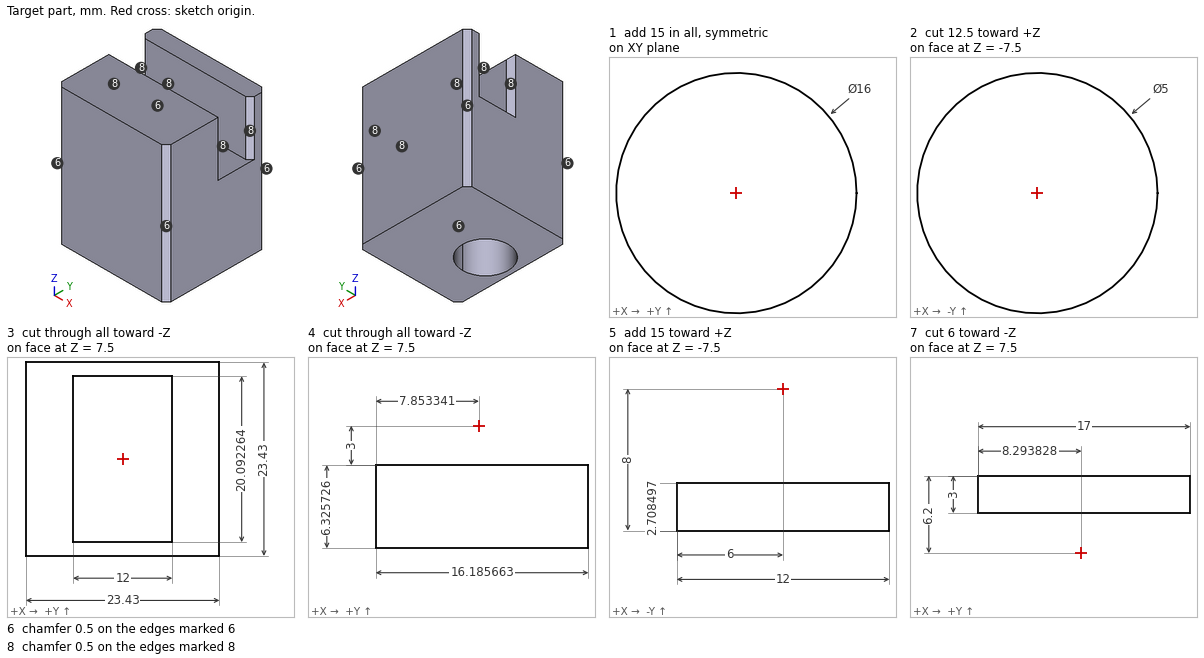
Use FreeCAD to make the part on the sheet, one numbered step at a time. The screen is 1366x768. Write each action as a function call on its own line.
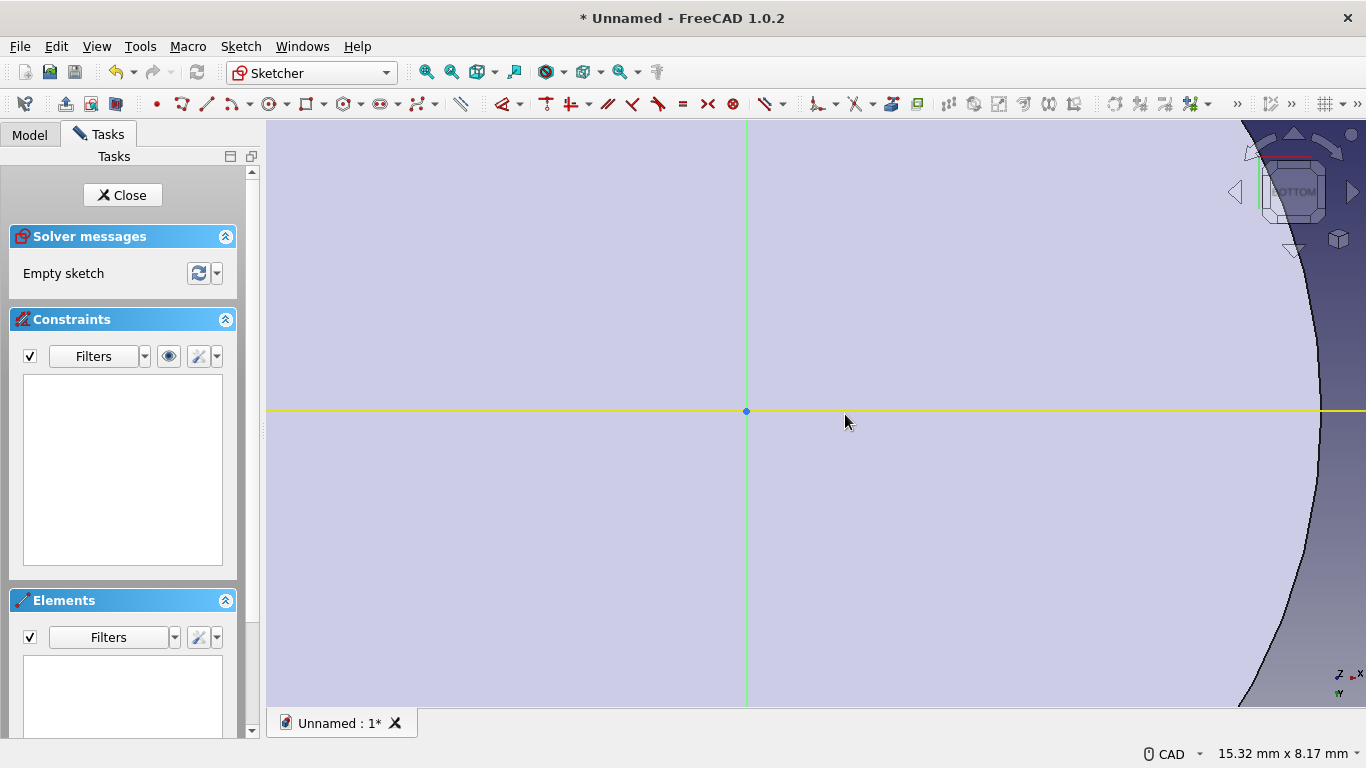
click(268, 104)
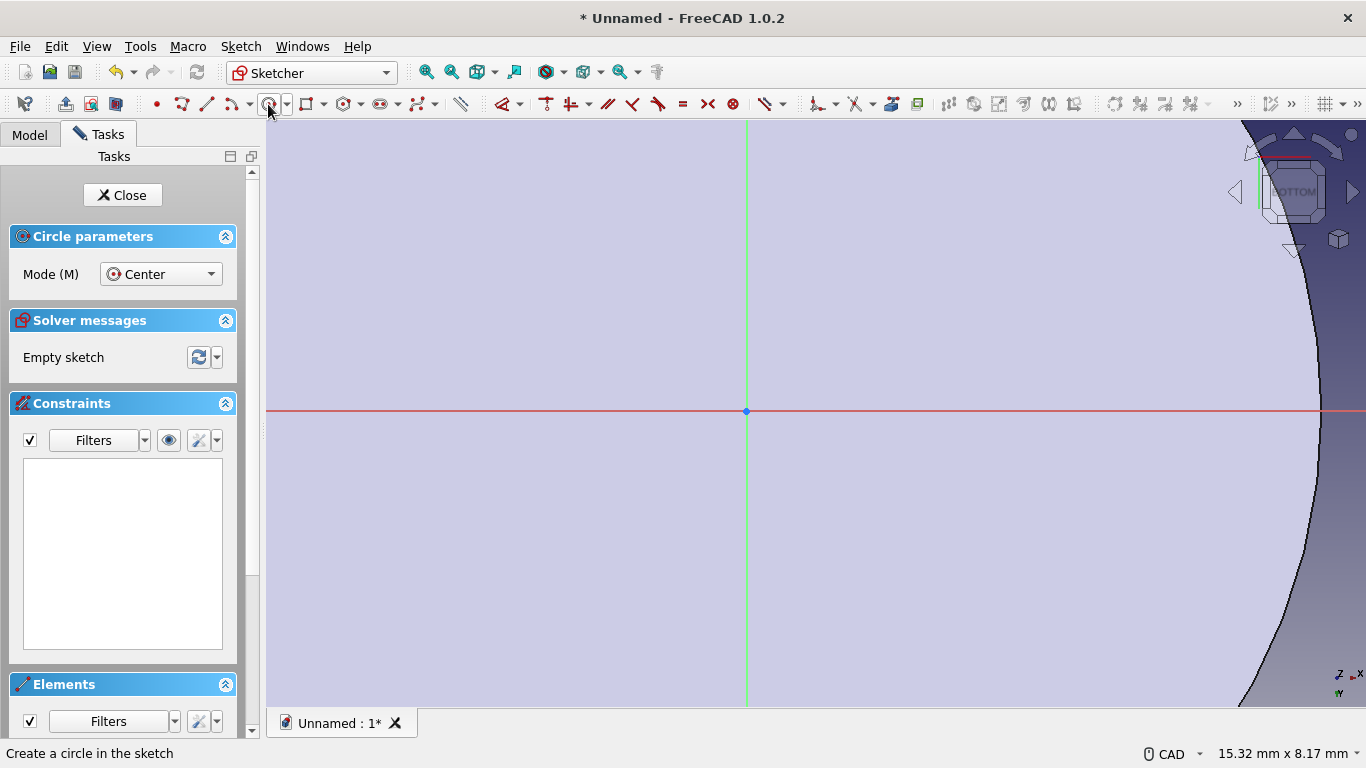
click(747, 411)
click(874, 284)
key(Escape)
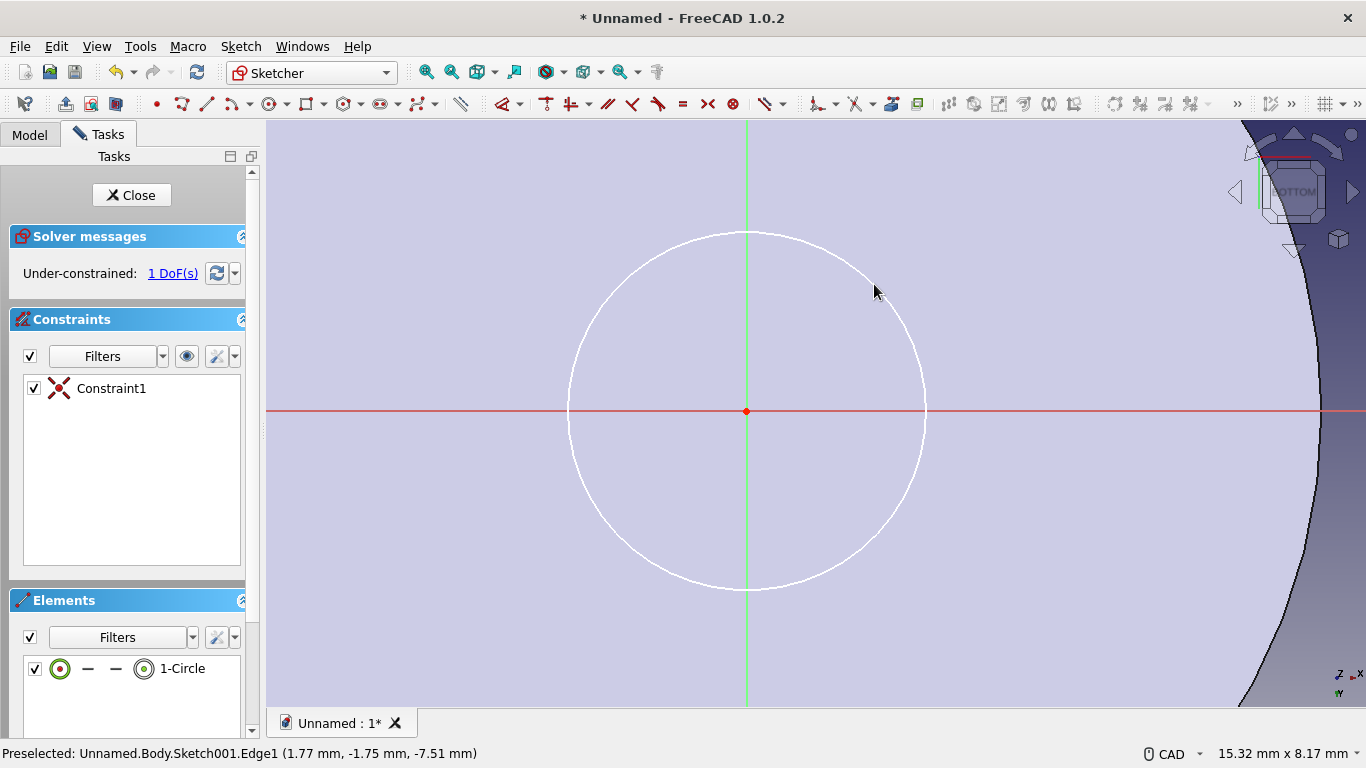
click(502, 104)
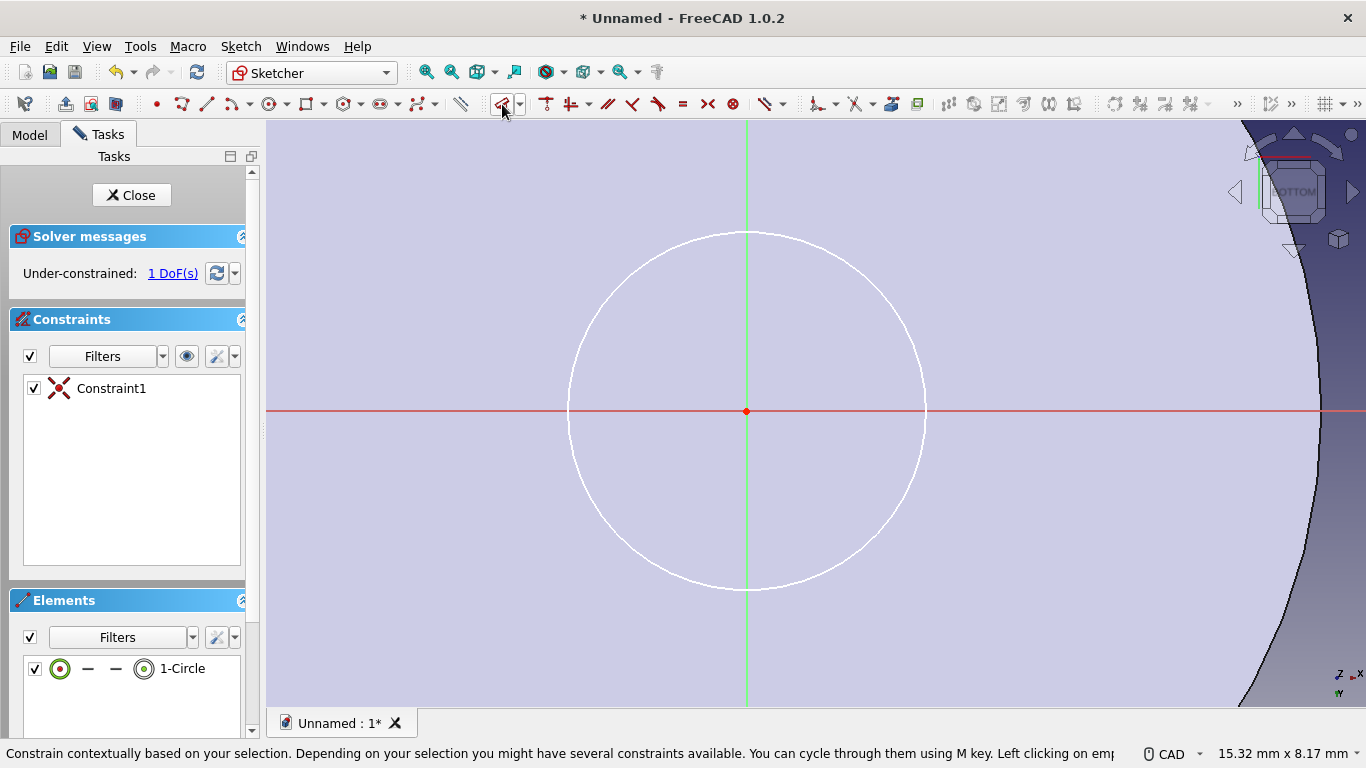
click(873, 284)
click(896, 261)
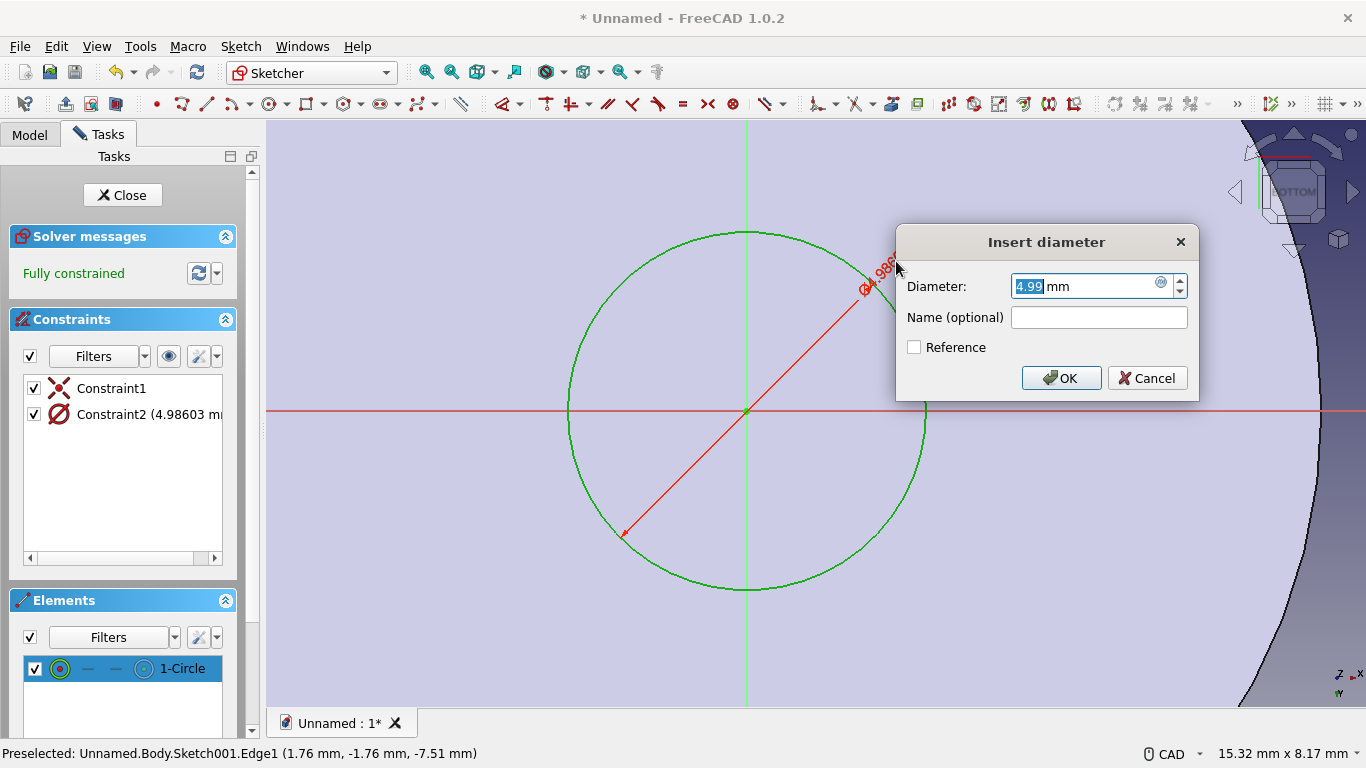
text(5)
key(Return)
key(Escape)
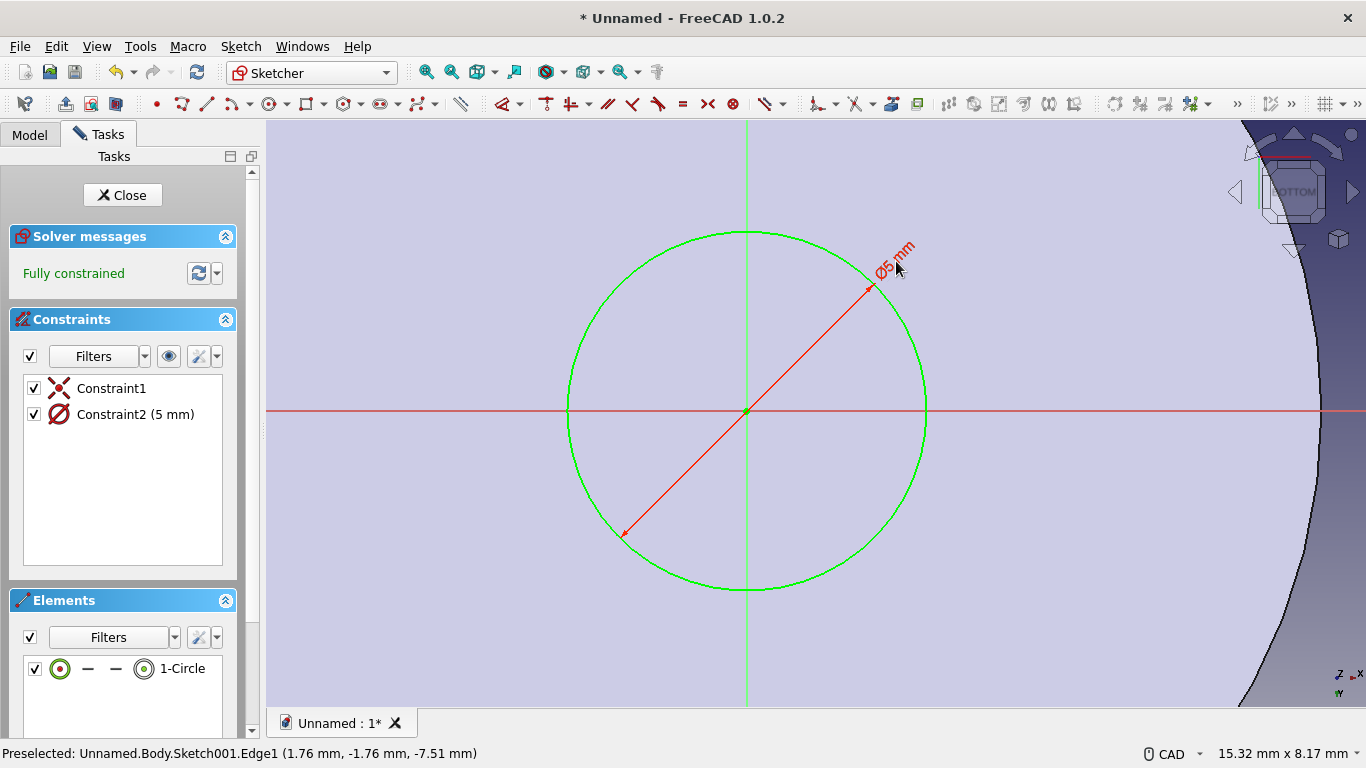
click(123, 195)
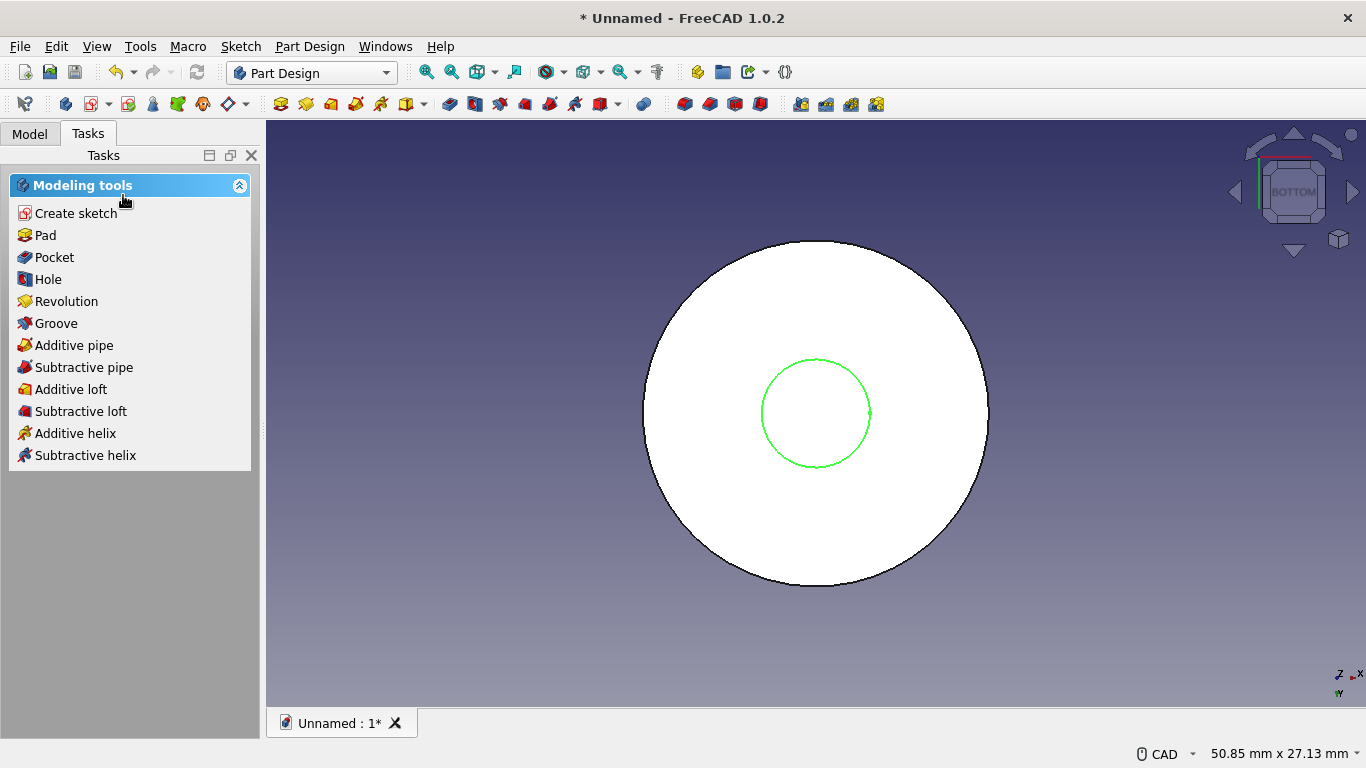
click(450, 104)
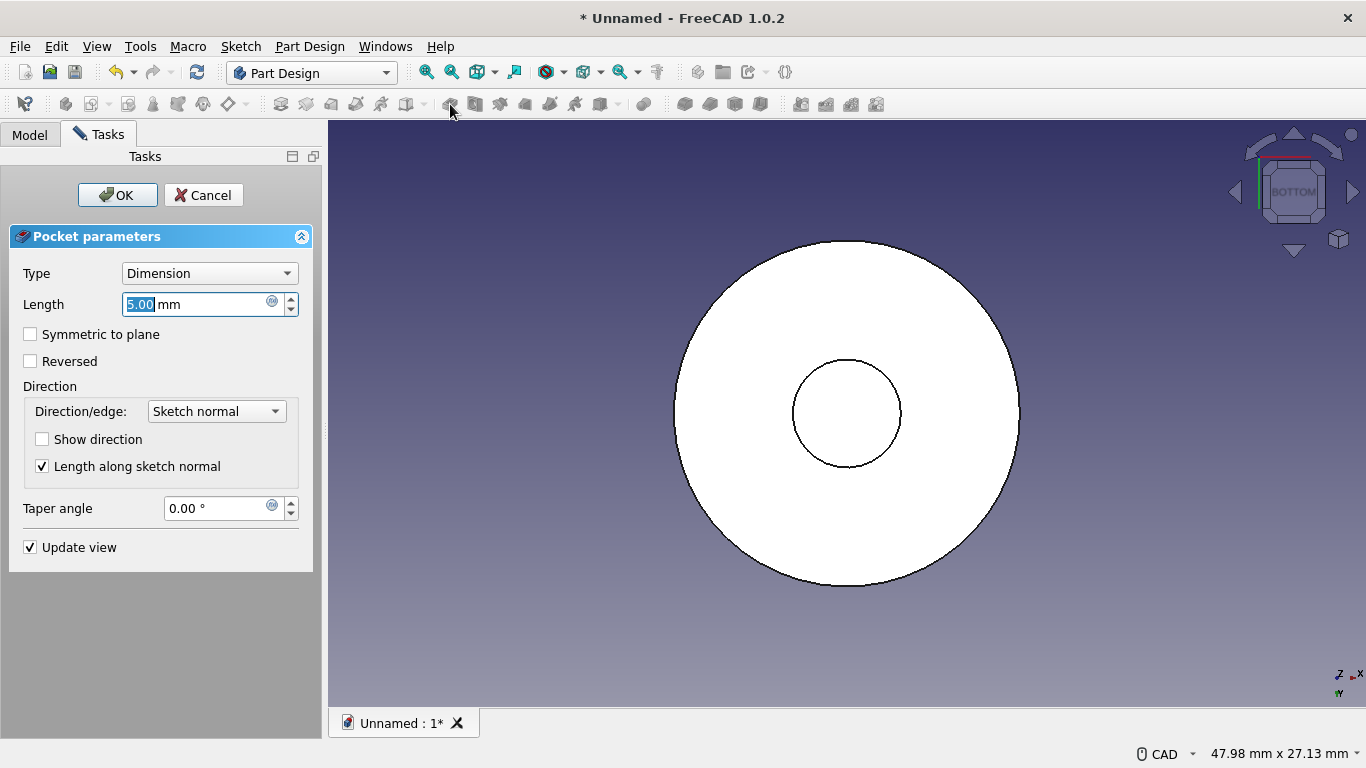
text(12.5)
key(Tab)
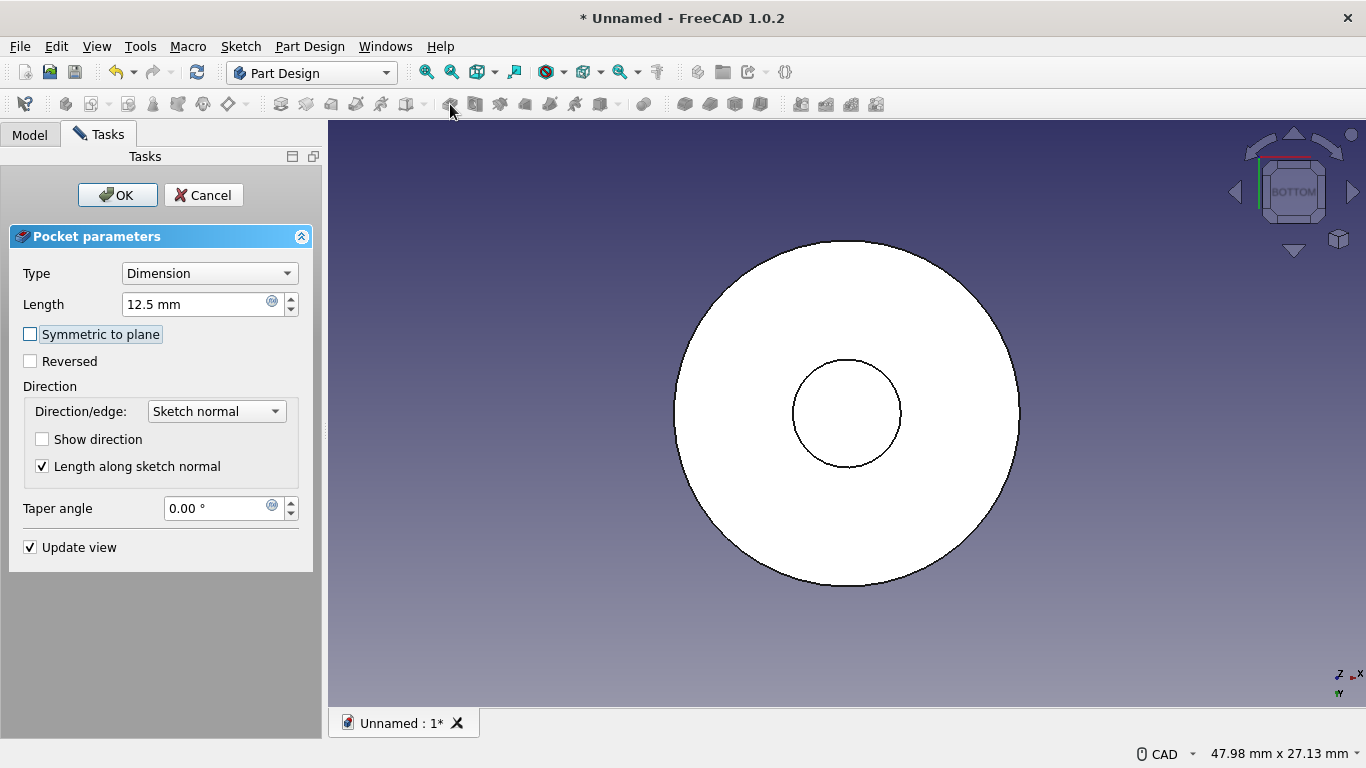
click(118, 195)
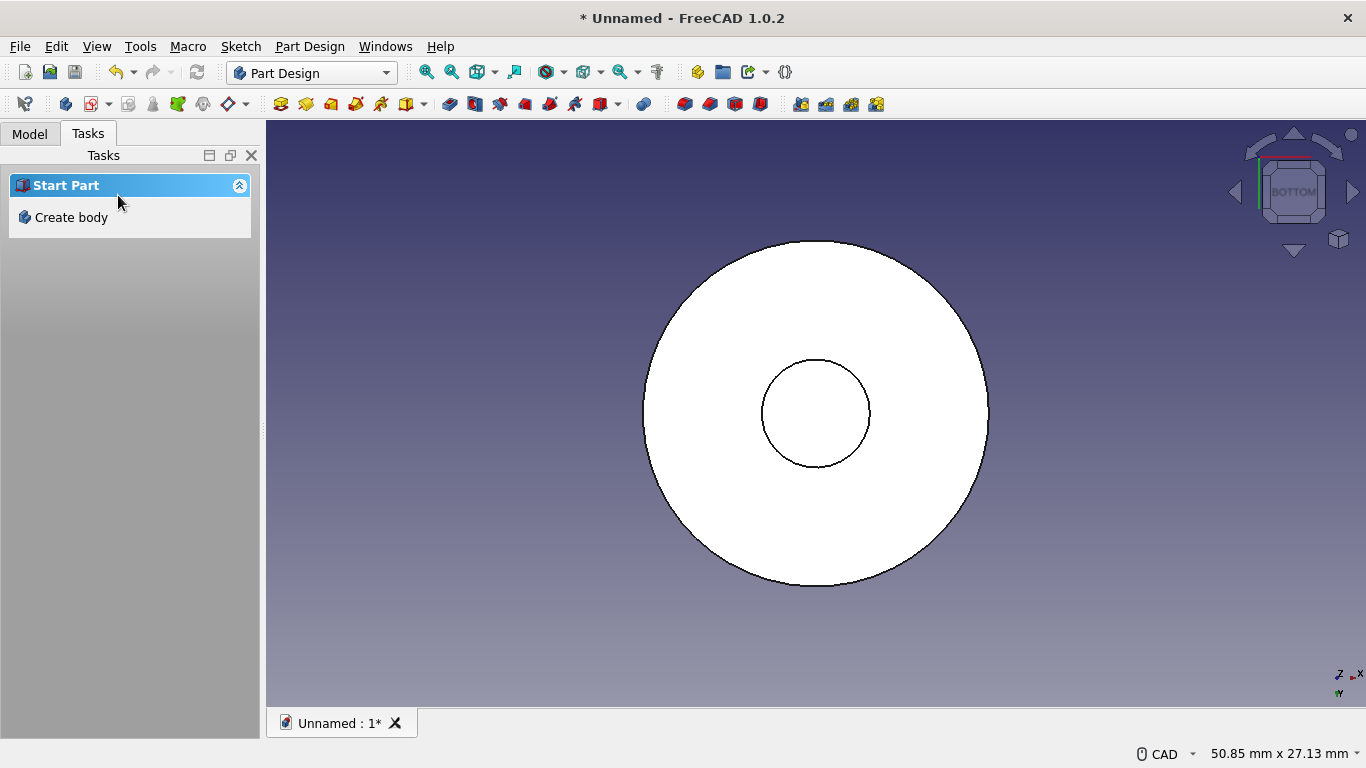
key(0)